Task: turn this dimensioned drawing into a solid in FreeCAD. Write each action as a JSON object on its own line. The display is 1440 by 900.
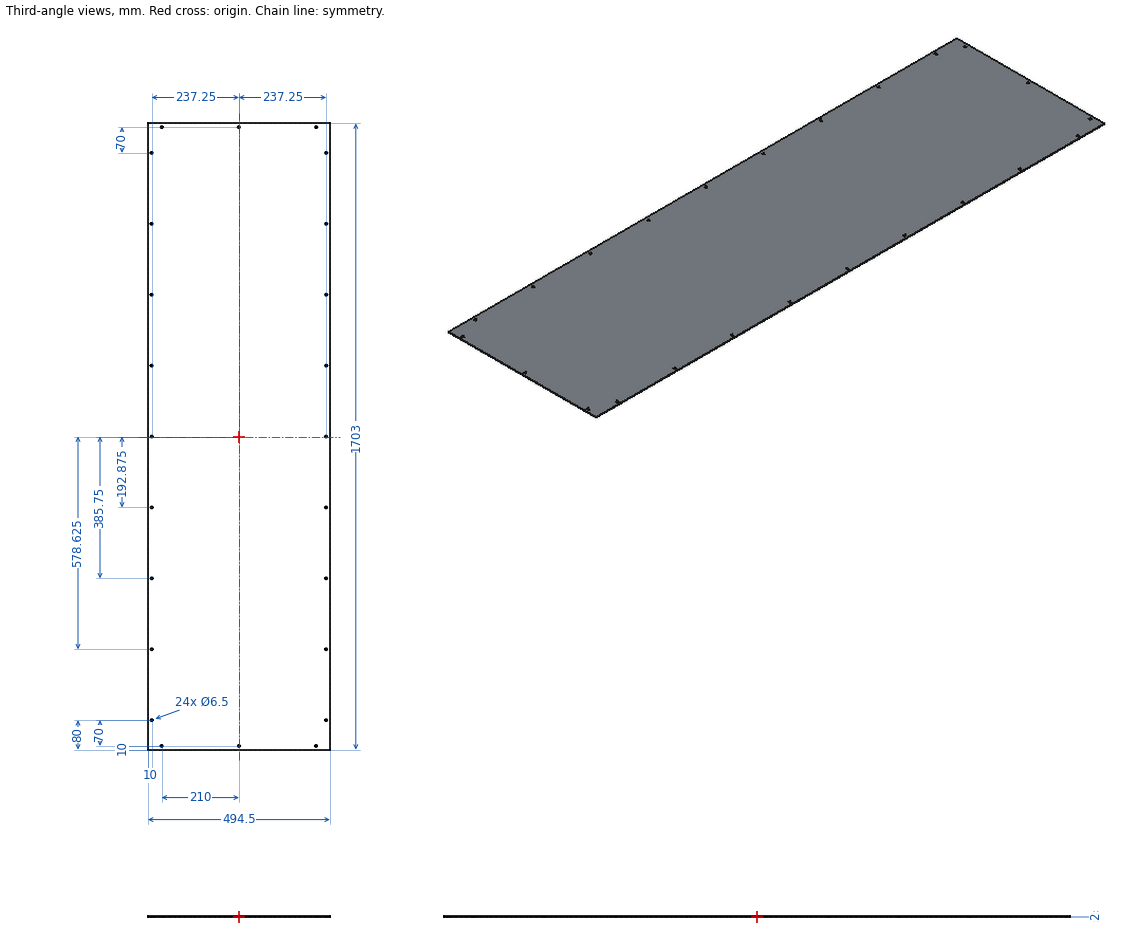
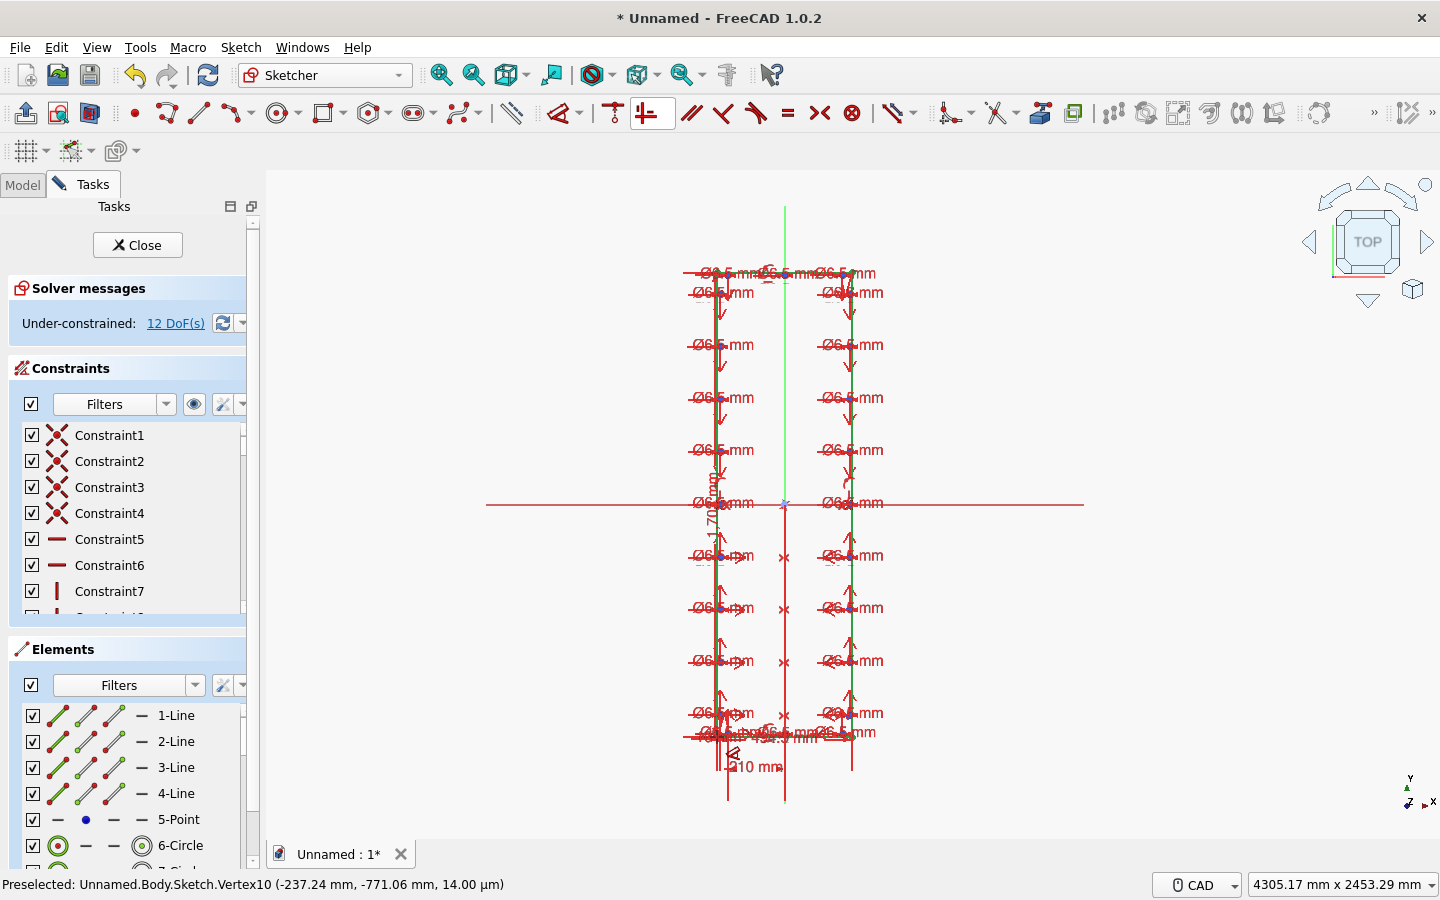
{"action": "scroll", "coordinate": [717, 737], "scroll_direction": "up", "scroll_amount": 3}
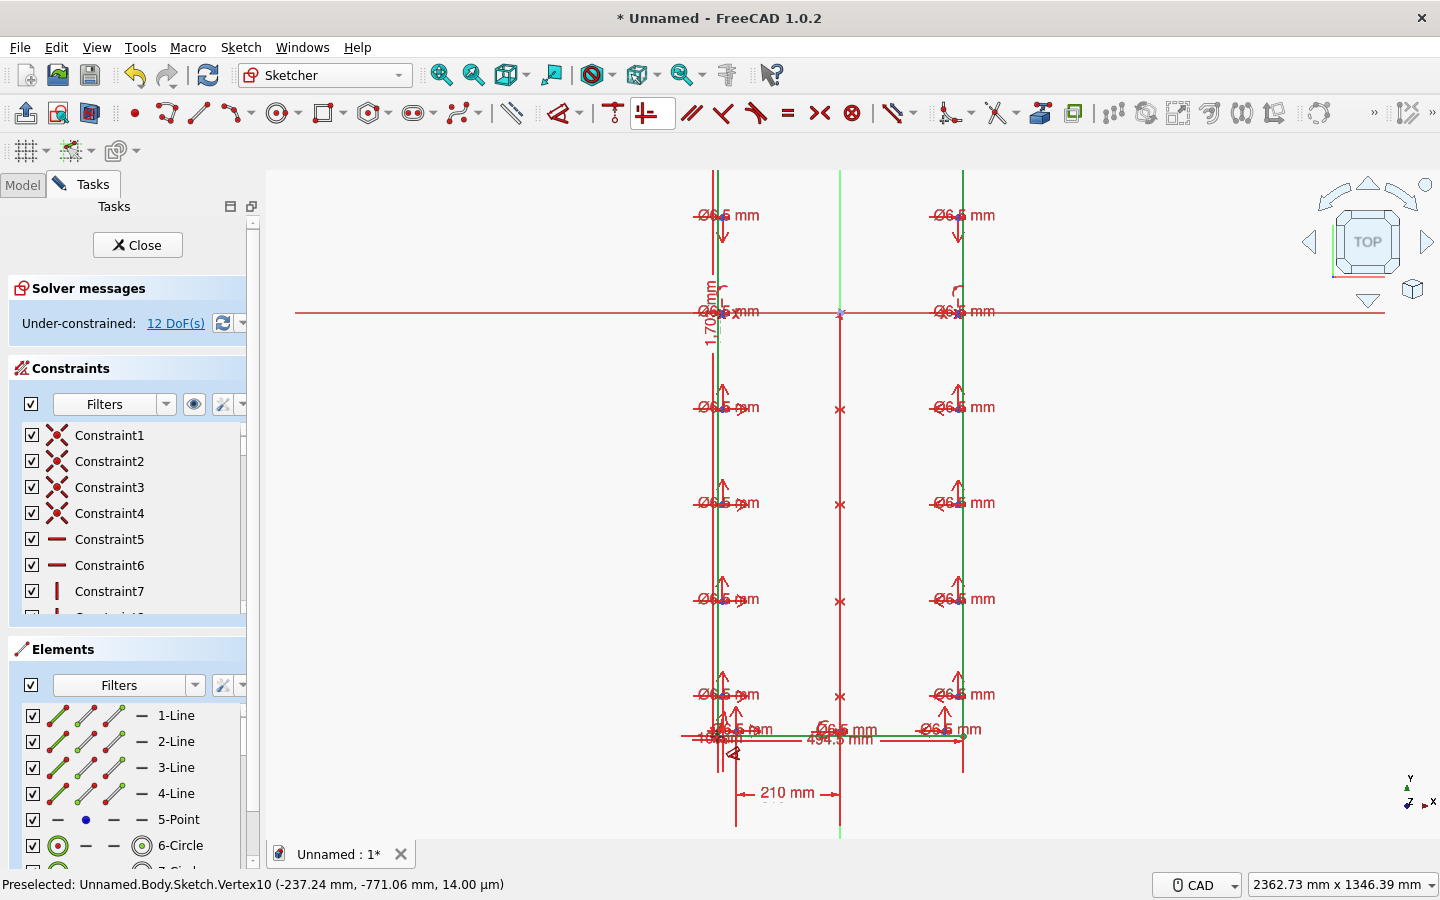
{"action": "left_click", "coordinate": [718, 736]}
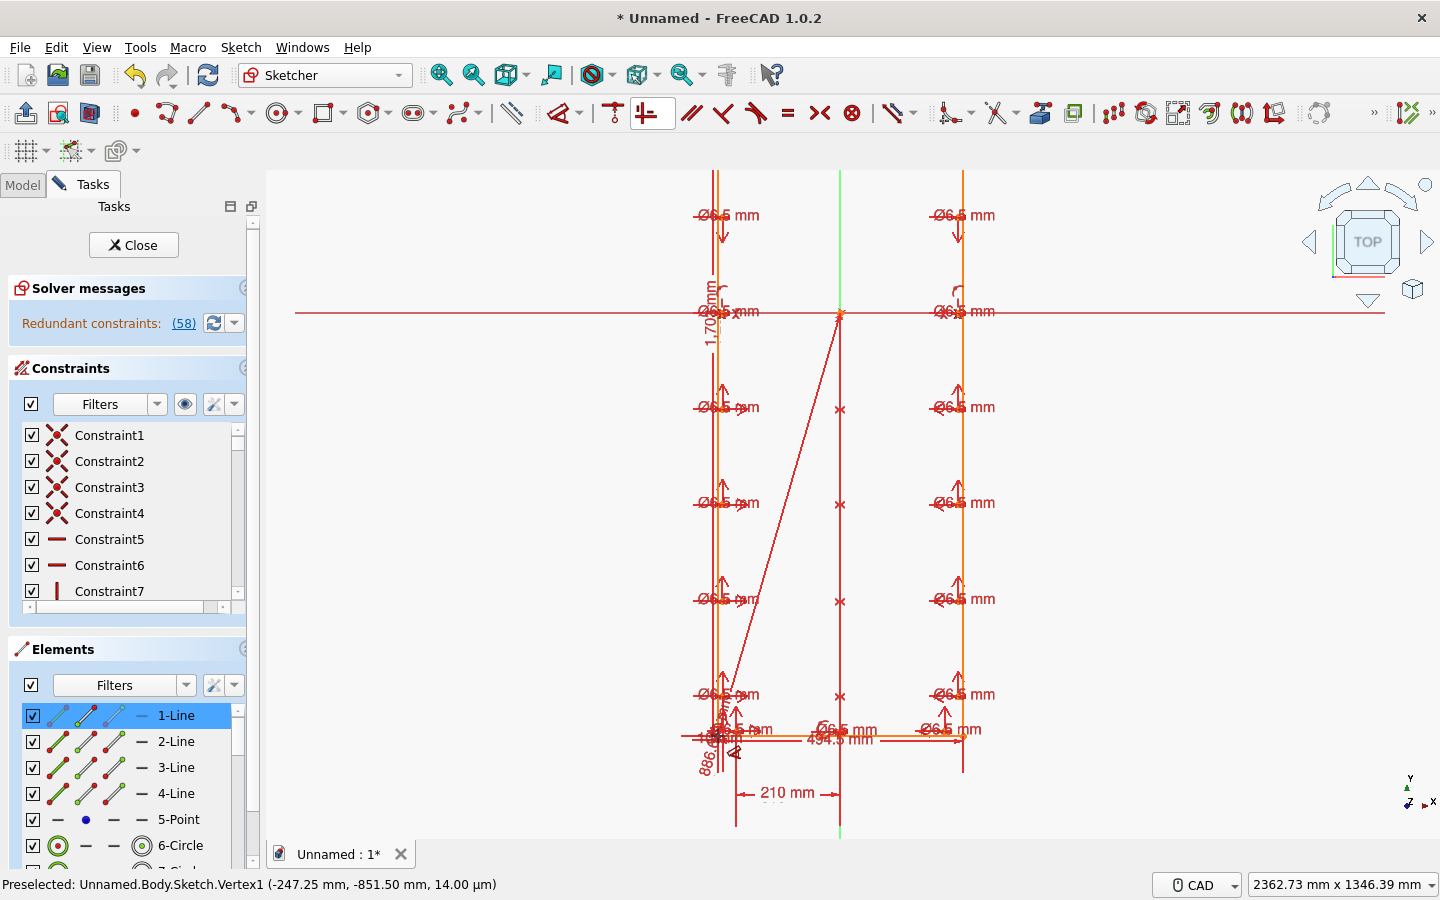
{"action": "left_click", "coordinate": [723, 696]}
{"action": "left_click", "coordinate": [684, 716]}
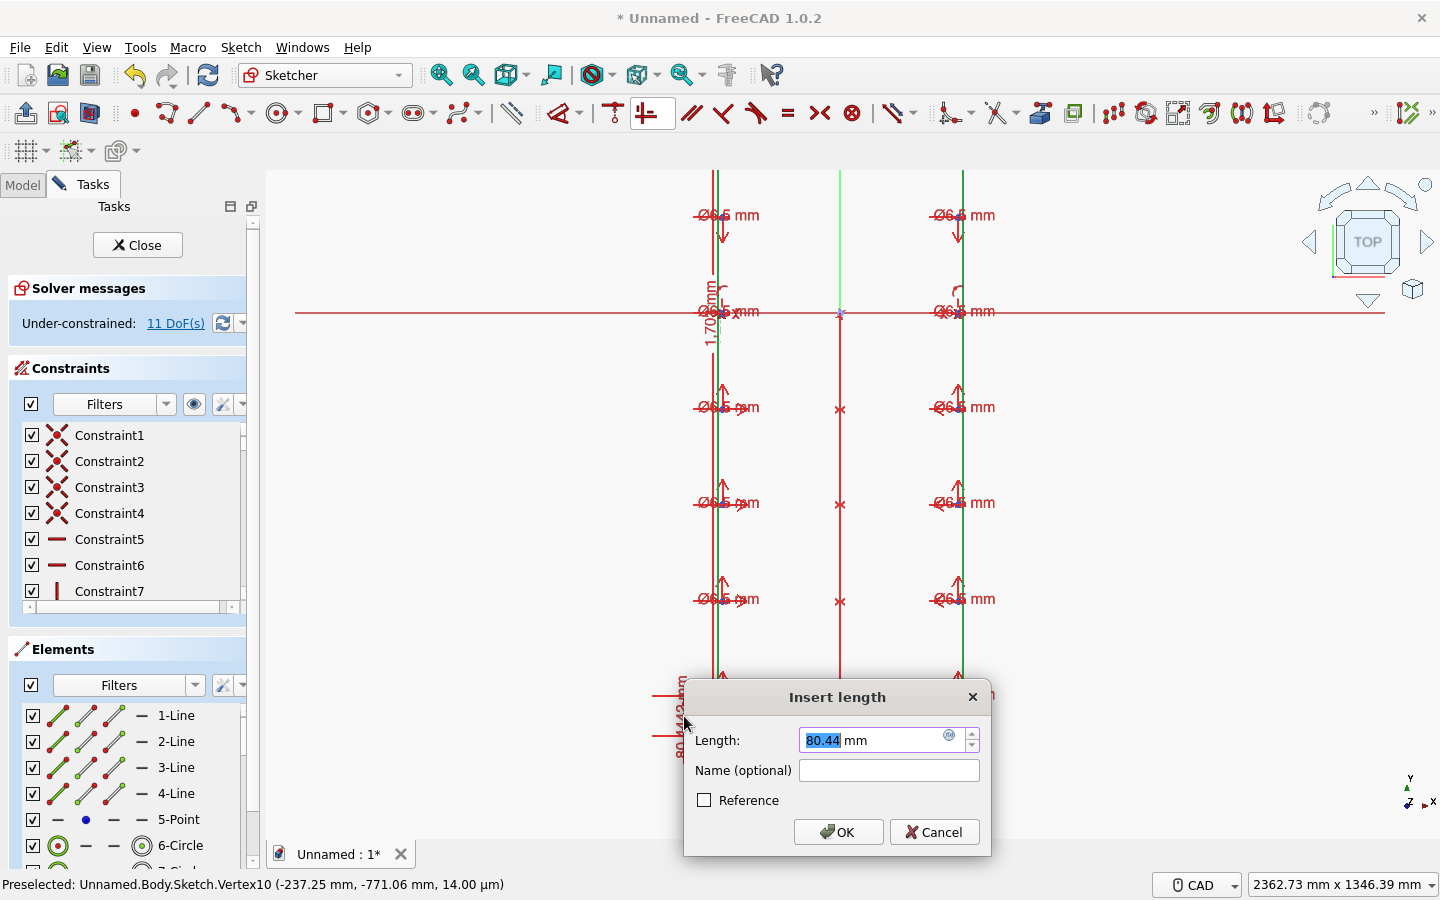
{"action": "type", "text": "80"}
{"action": "key", "text": "Return"}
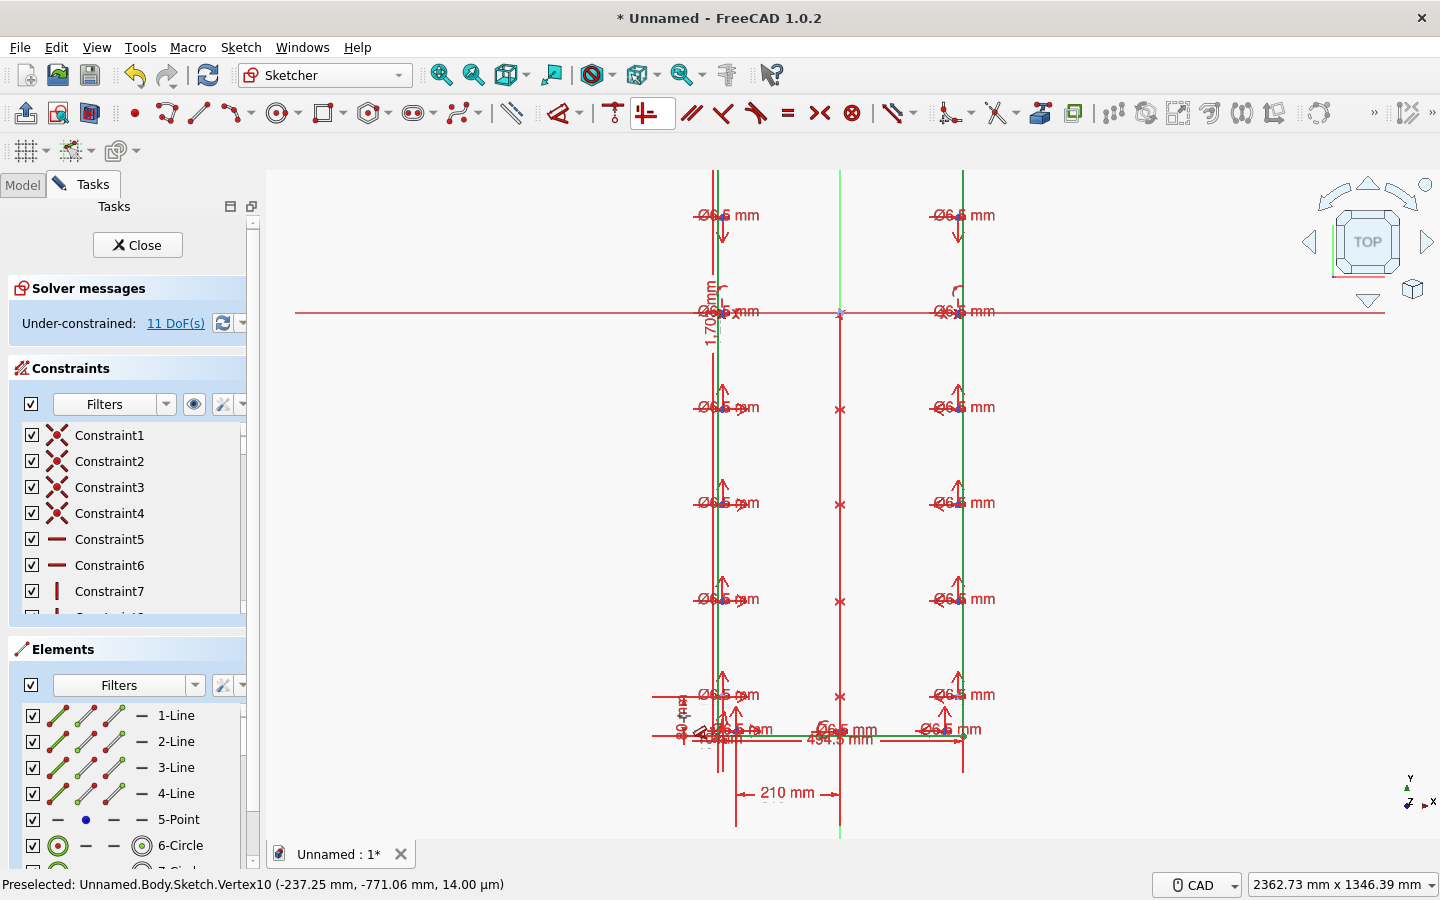
{"action": "scroll", "coordinate": [718, 736], "scroll_direction": "up", "scroll_amount": 11}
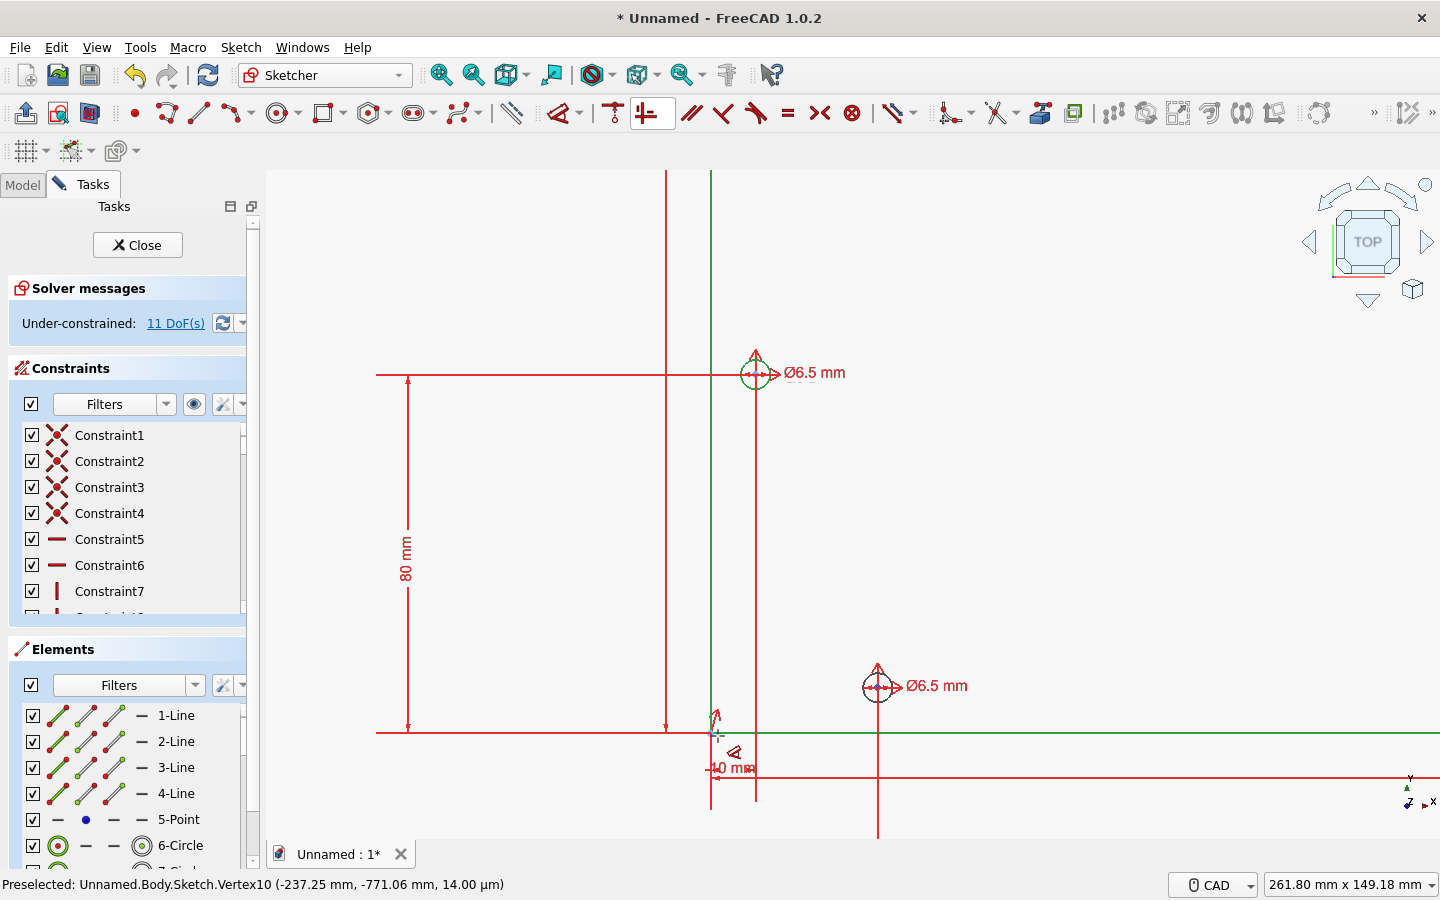
{"action": "left_click", "coordinate": [711, 733]}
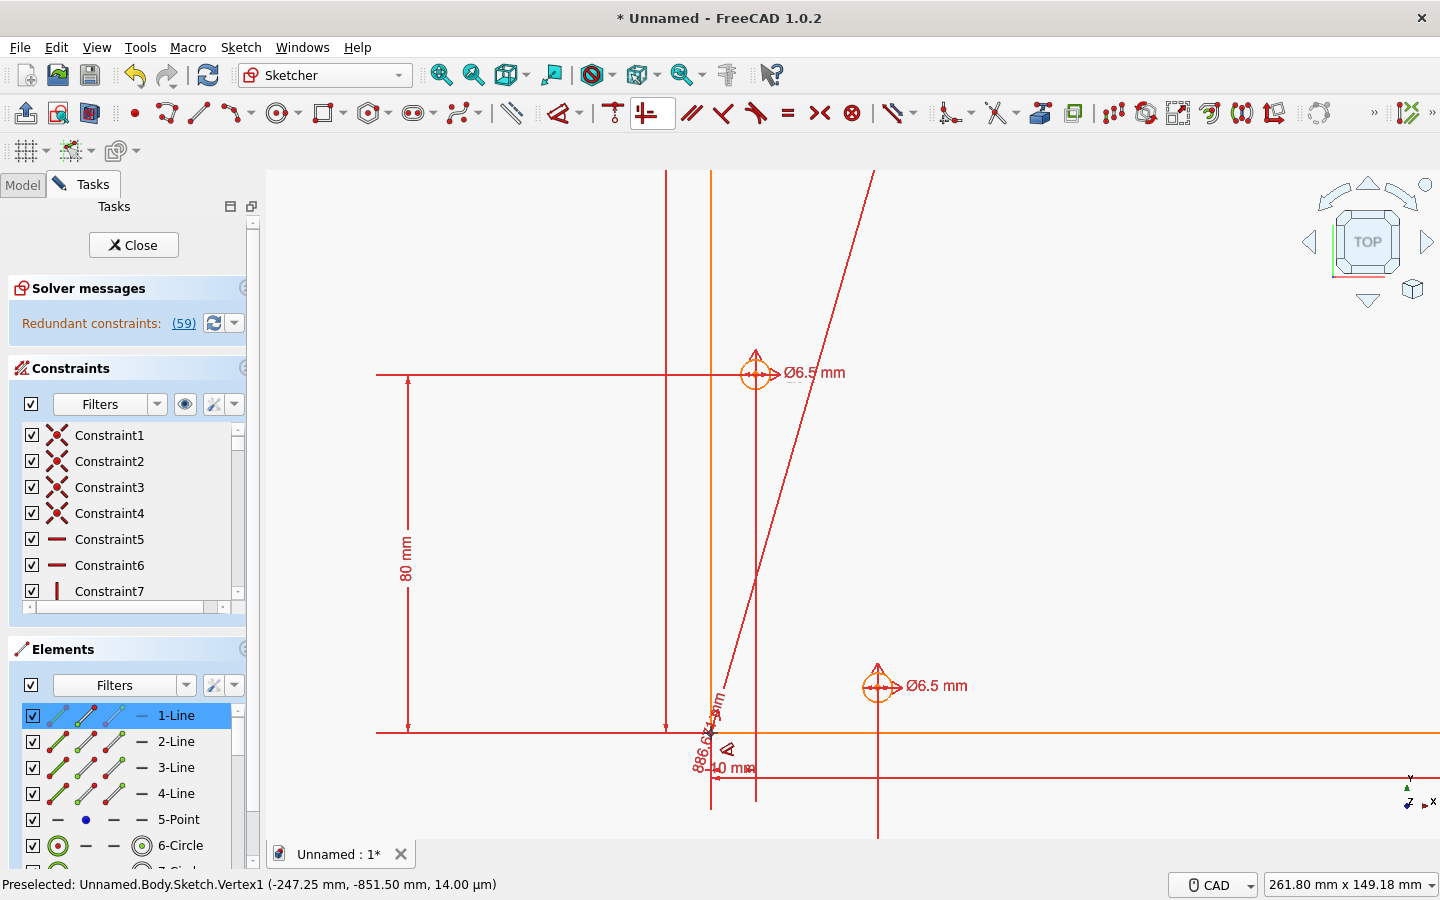
{"action": "left_click", "coordinate": [878, 688]}
{"action": "left_click", "coordinate": [677, 711]}